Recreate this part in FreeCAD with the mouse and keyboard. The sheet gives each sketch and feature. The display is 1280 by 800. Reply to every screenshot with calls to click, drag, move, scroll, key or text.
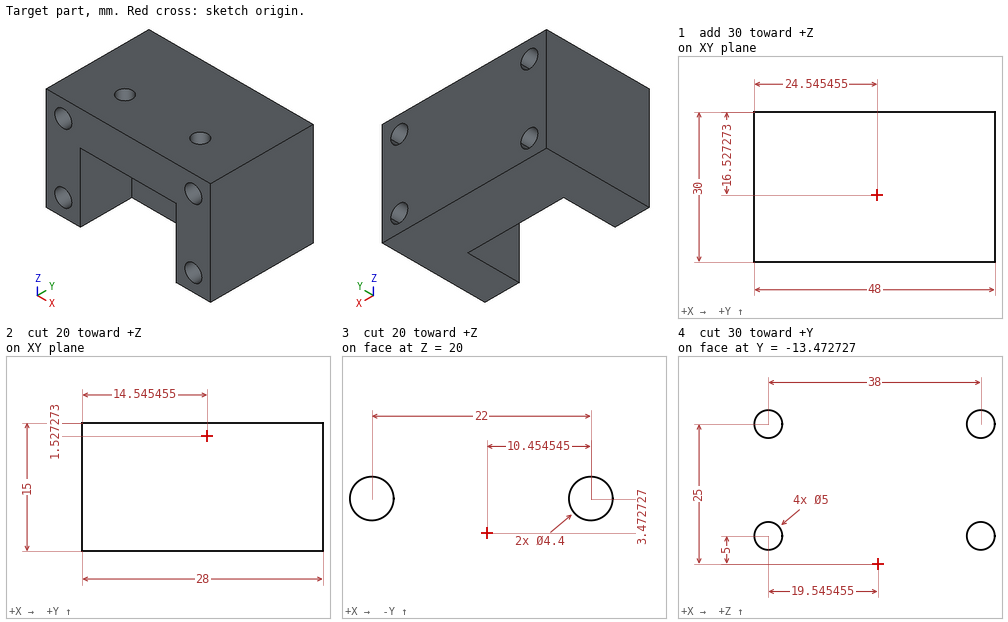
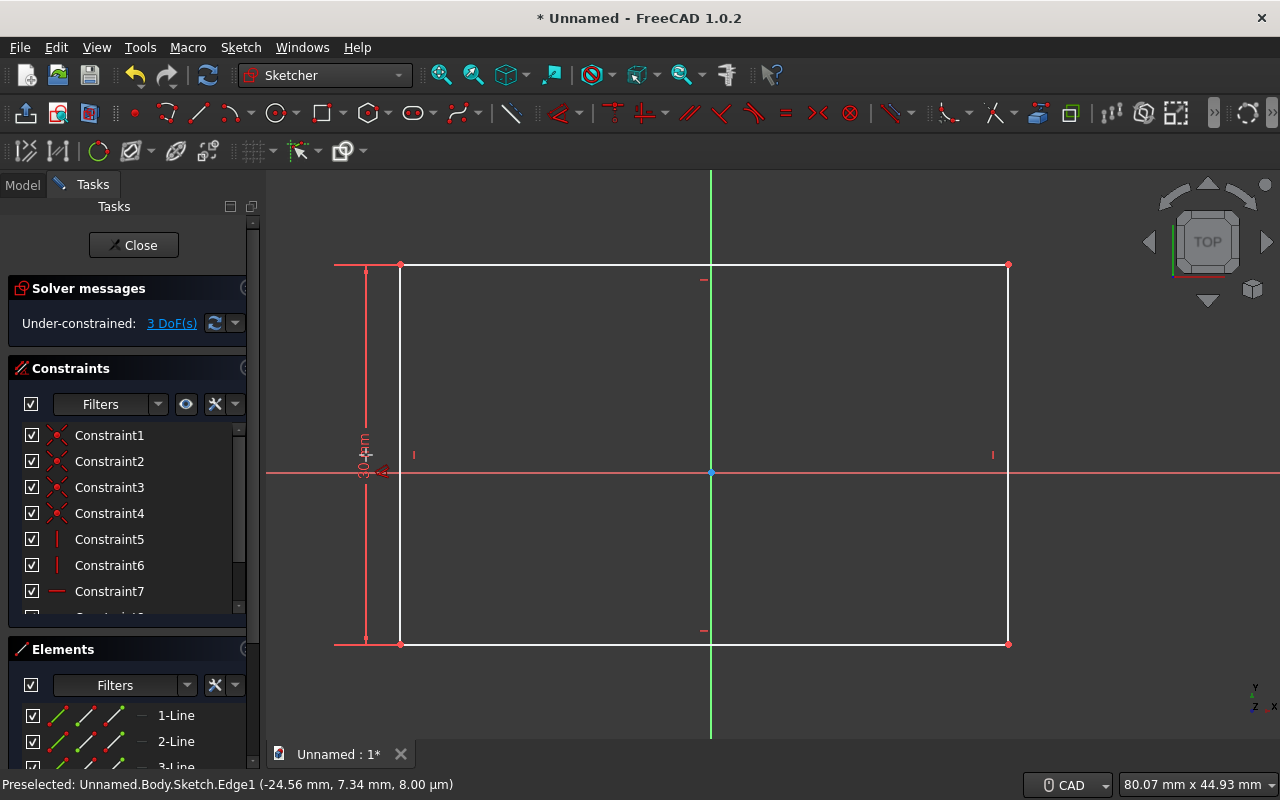
click(582, 645)
click(564, 679)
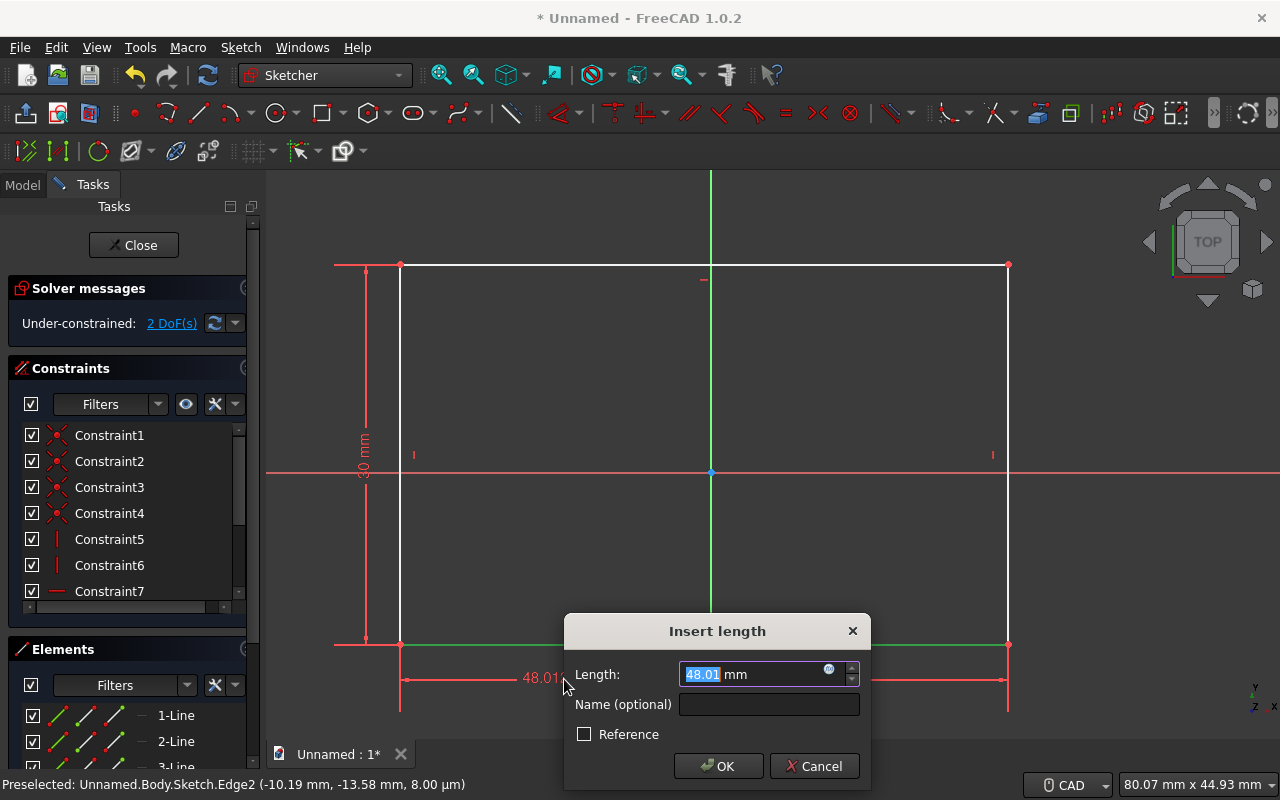
text(48)
key(Return)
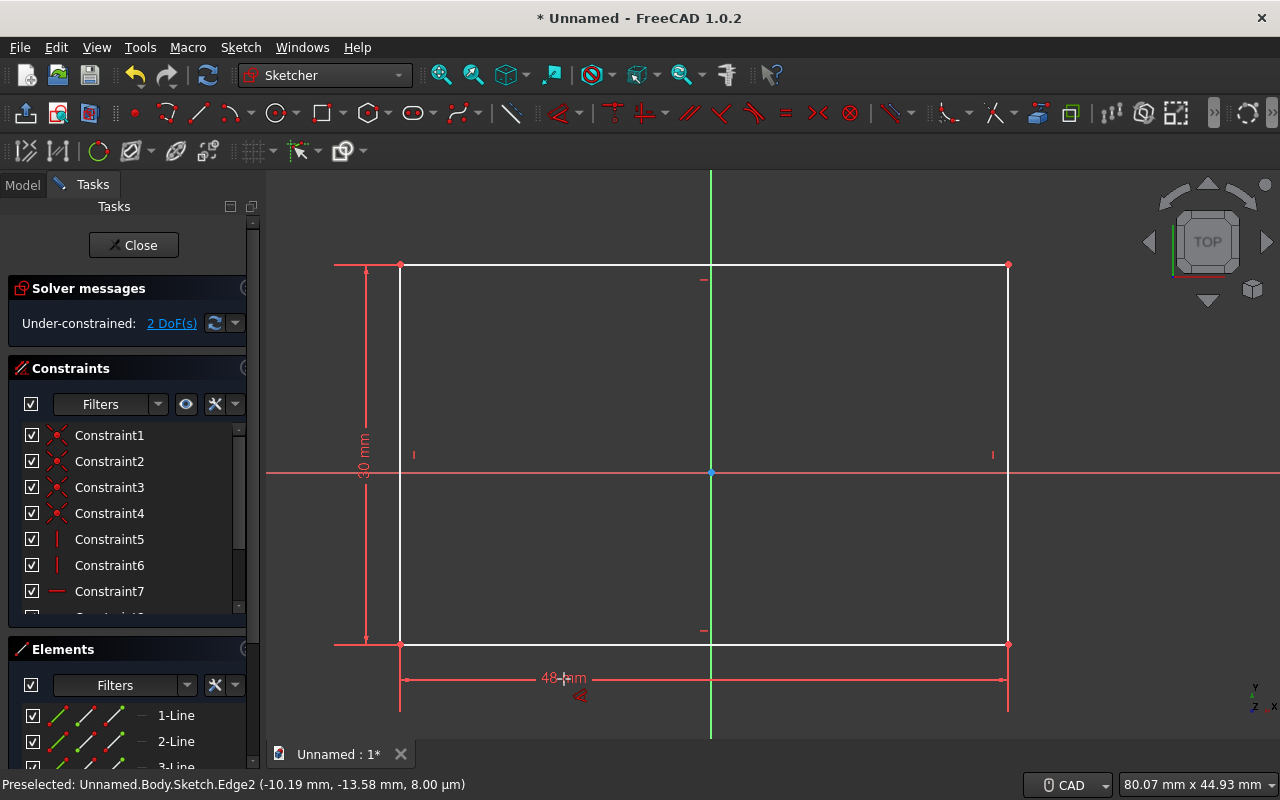
click(400, 265)
click(556, 231)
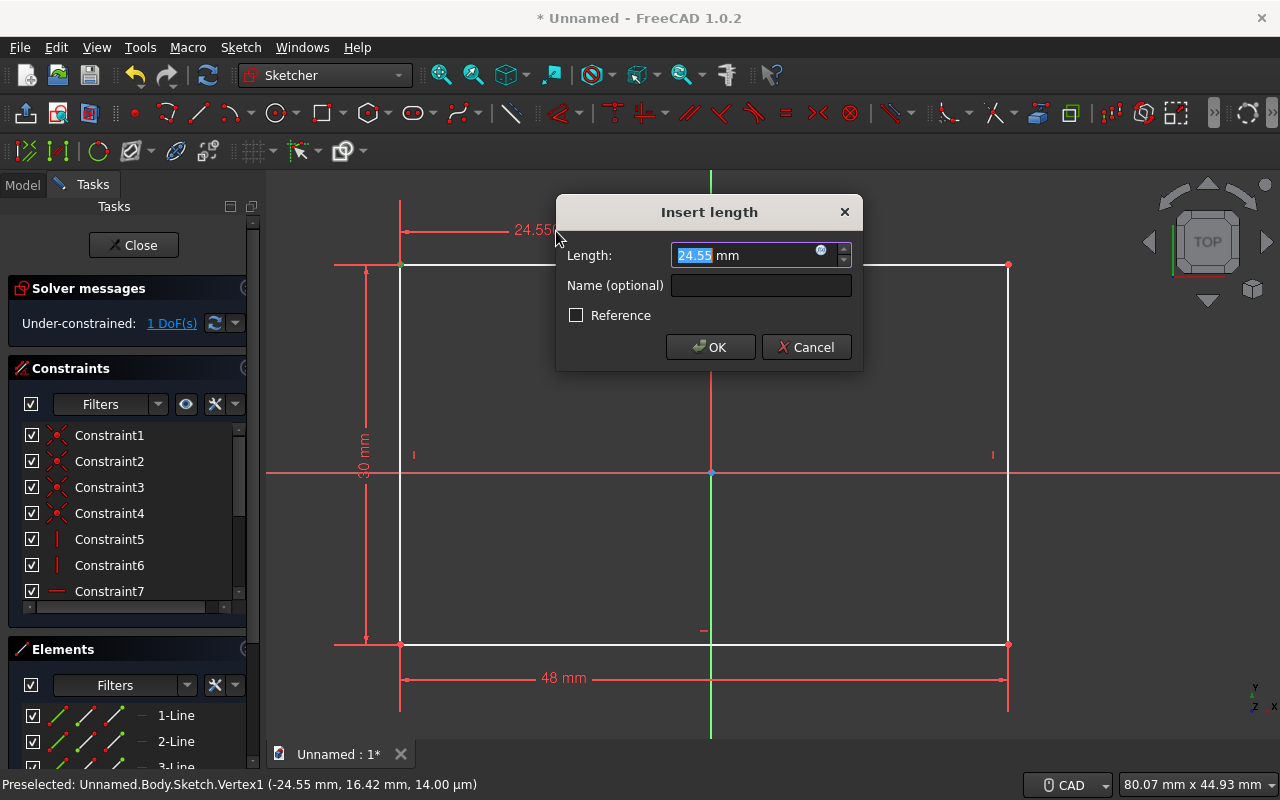
text(24.545455)
key(Return)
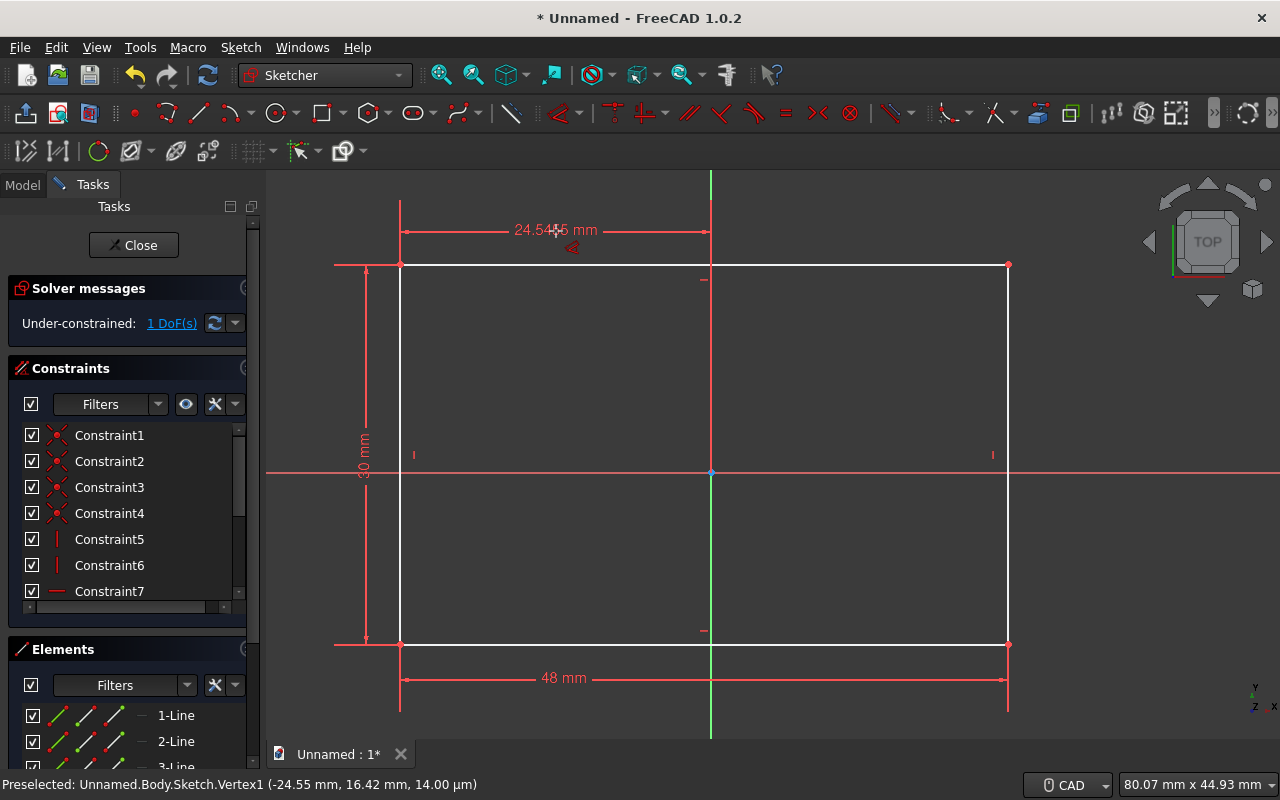
click(400, 265)
click(366, 369)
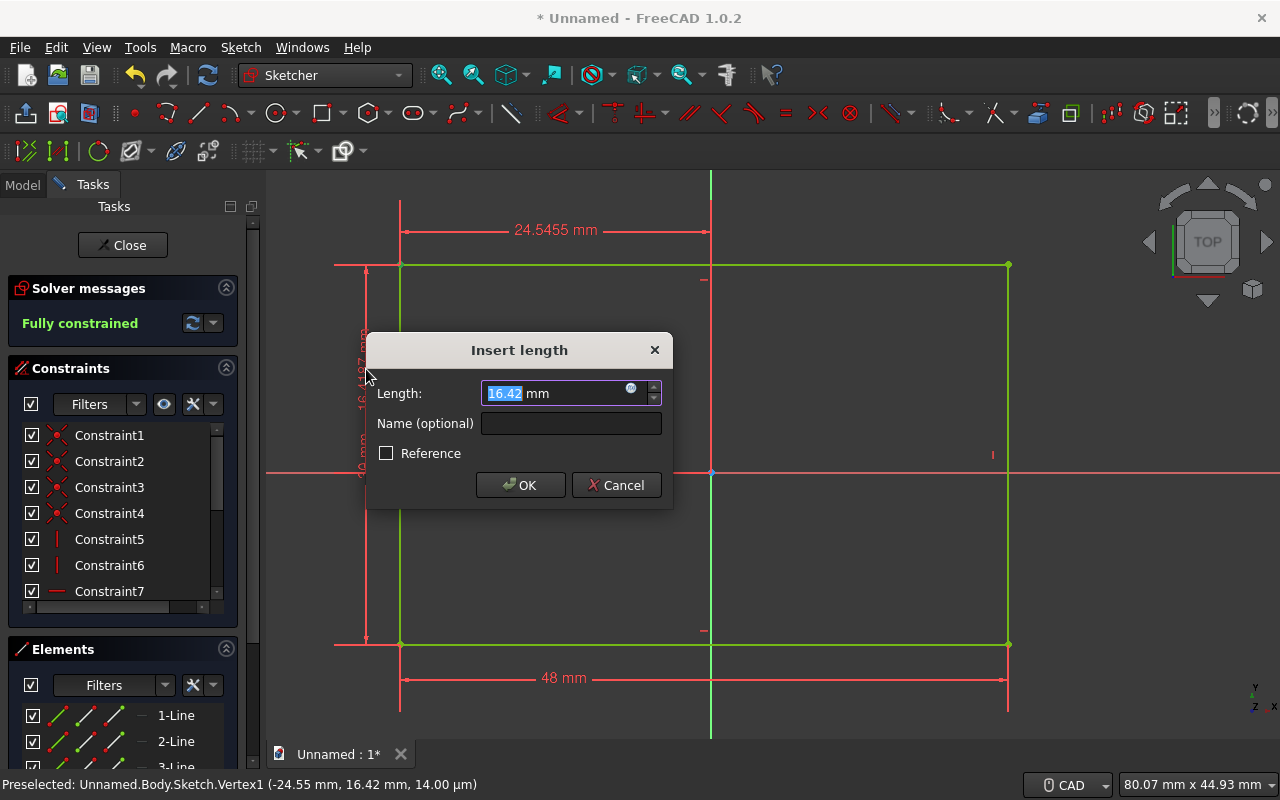
text(16.527273)
key(Return)
key(Escape)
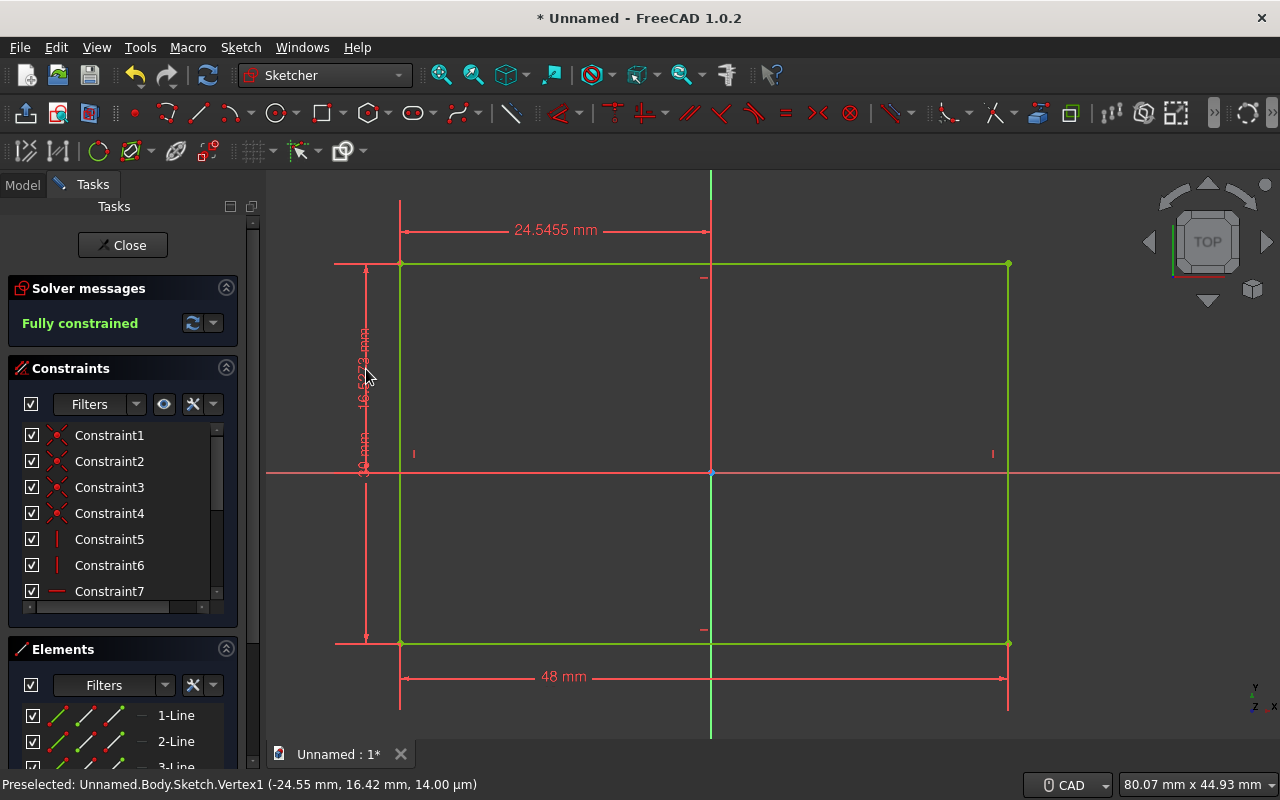
click(123, 245)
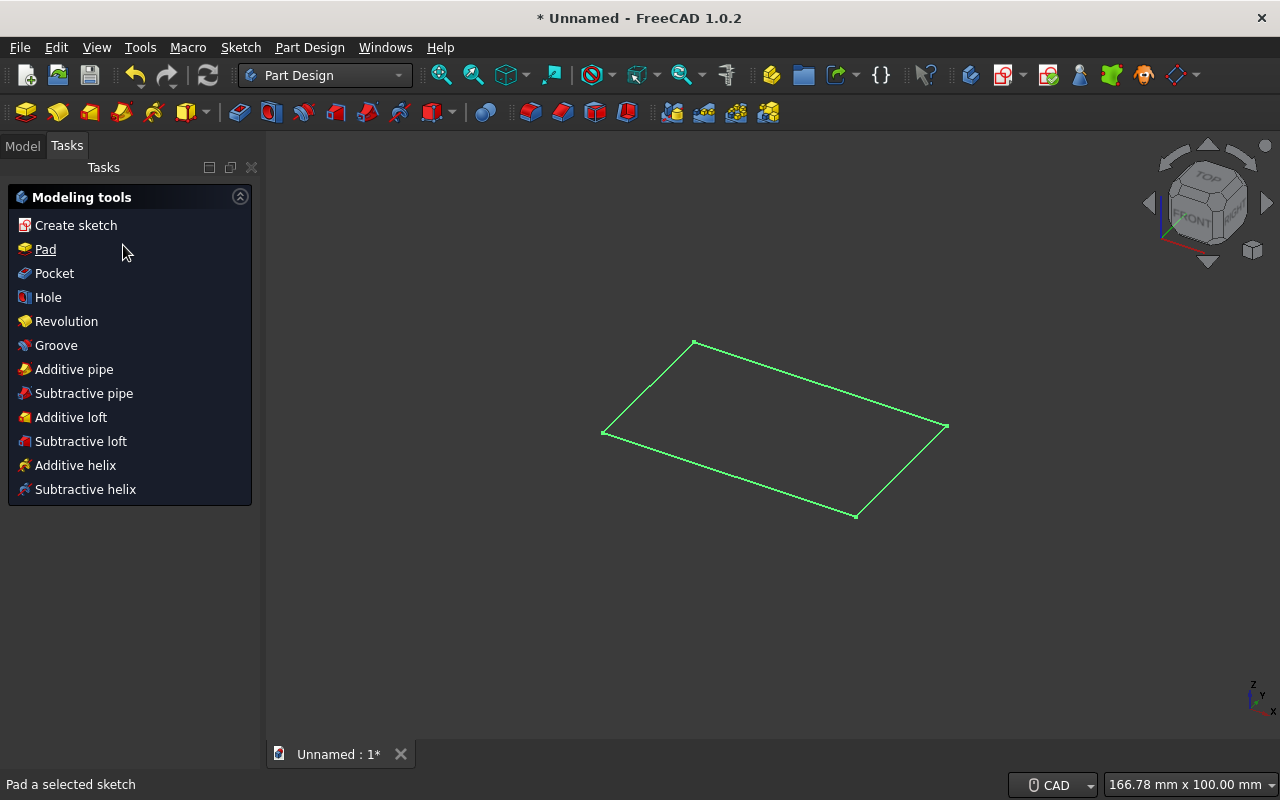
click(26, 112)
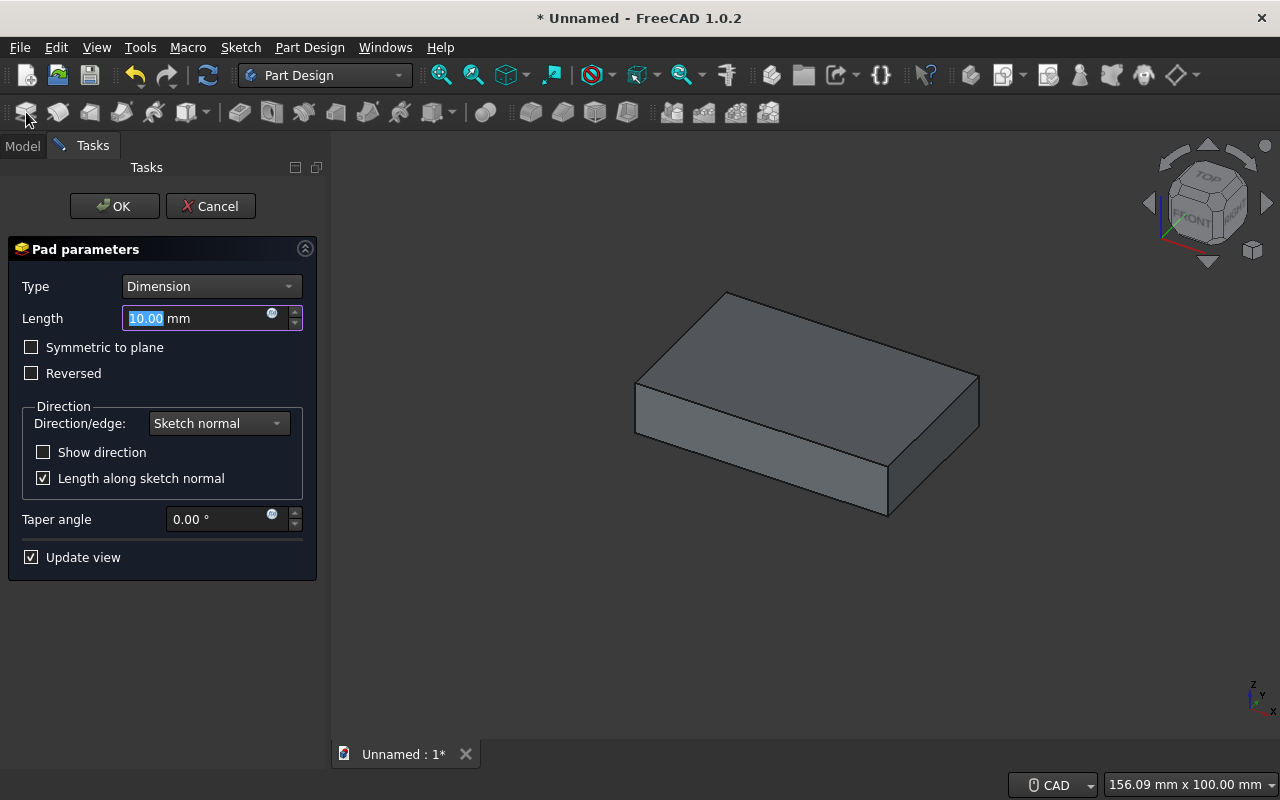
text(30)
key(Tab)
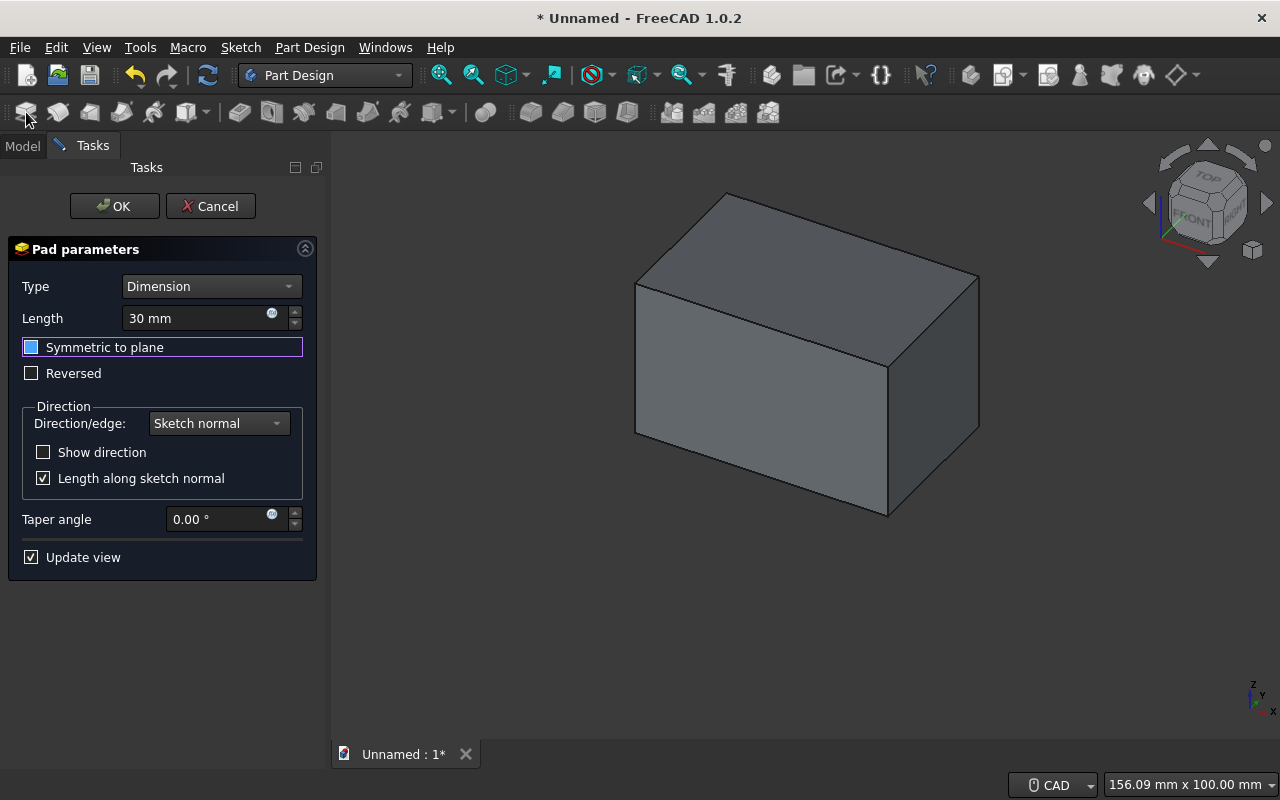
click(115, 206)